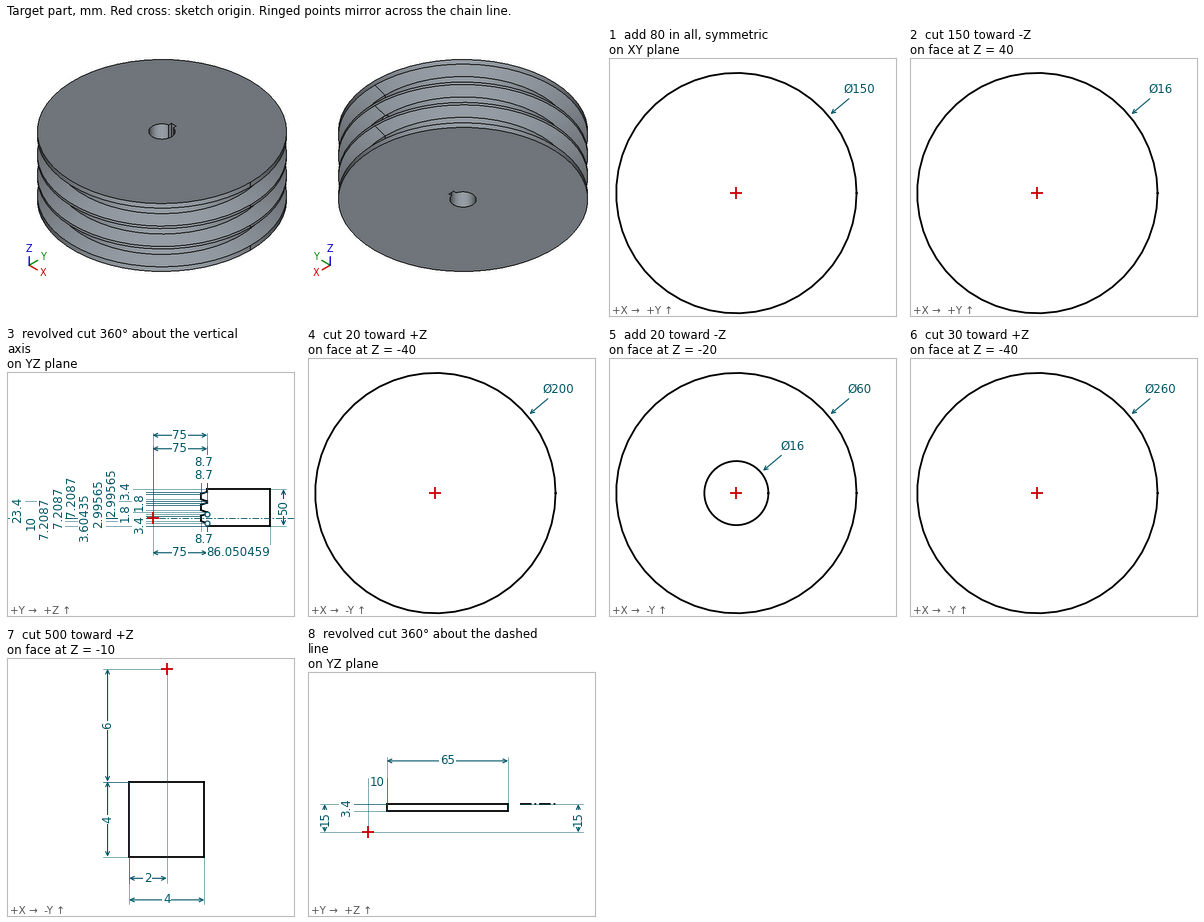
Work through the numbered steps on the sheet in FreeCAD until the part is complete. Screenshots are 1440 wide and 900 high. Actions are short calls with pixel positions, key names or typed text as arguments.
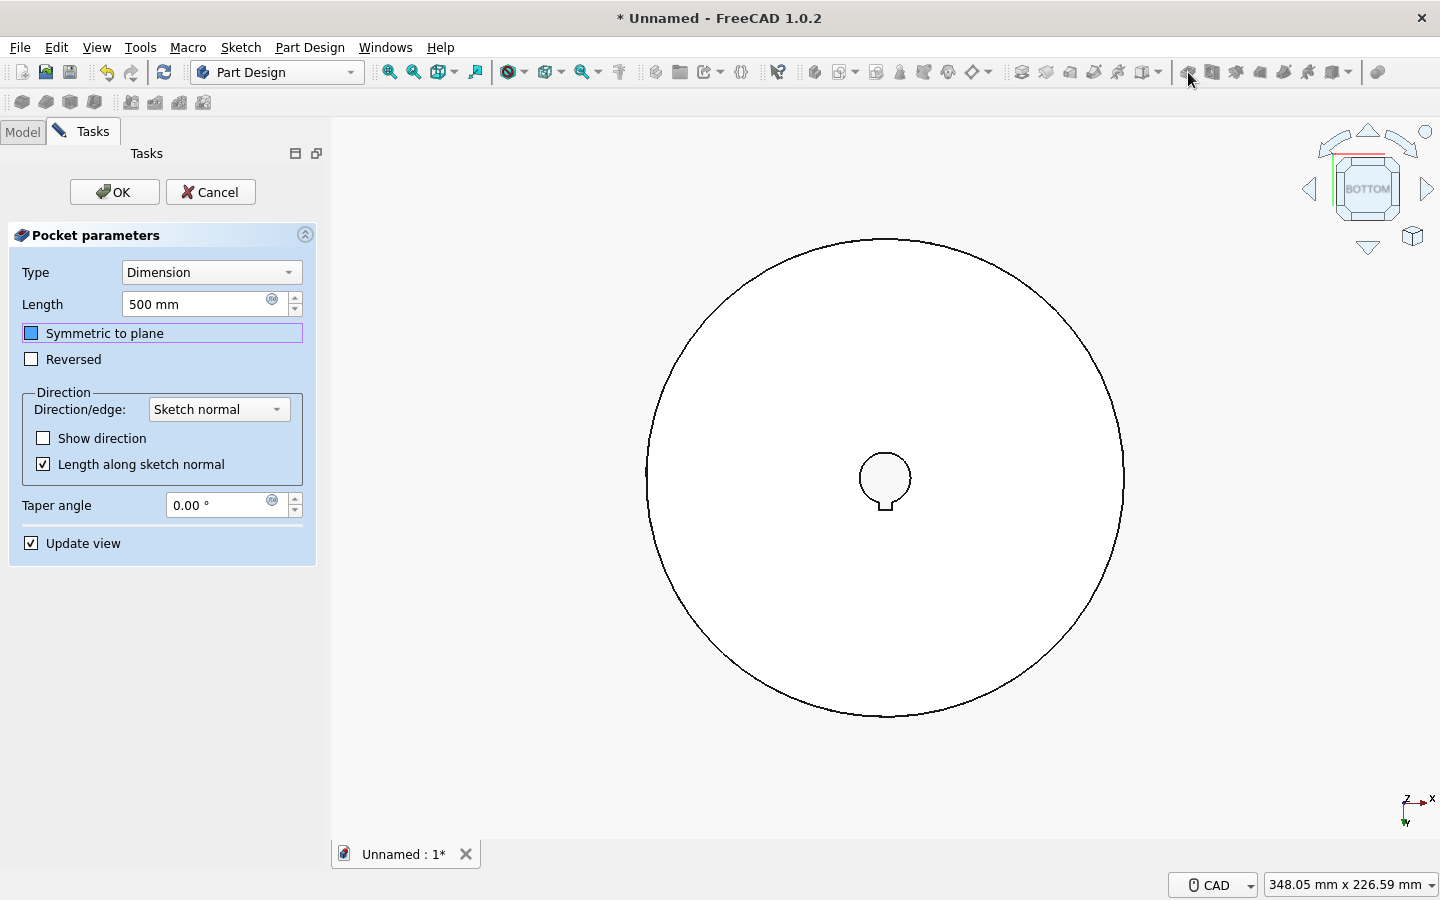
click(115, 192)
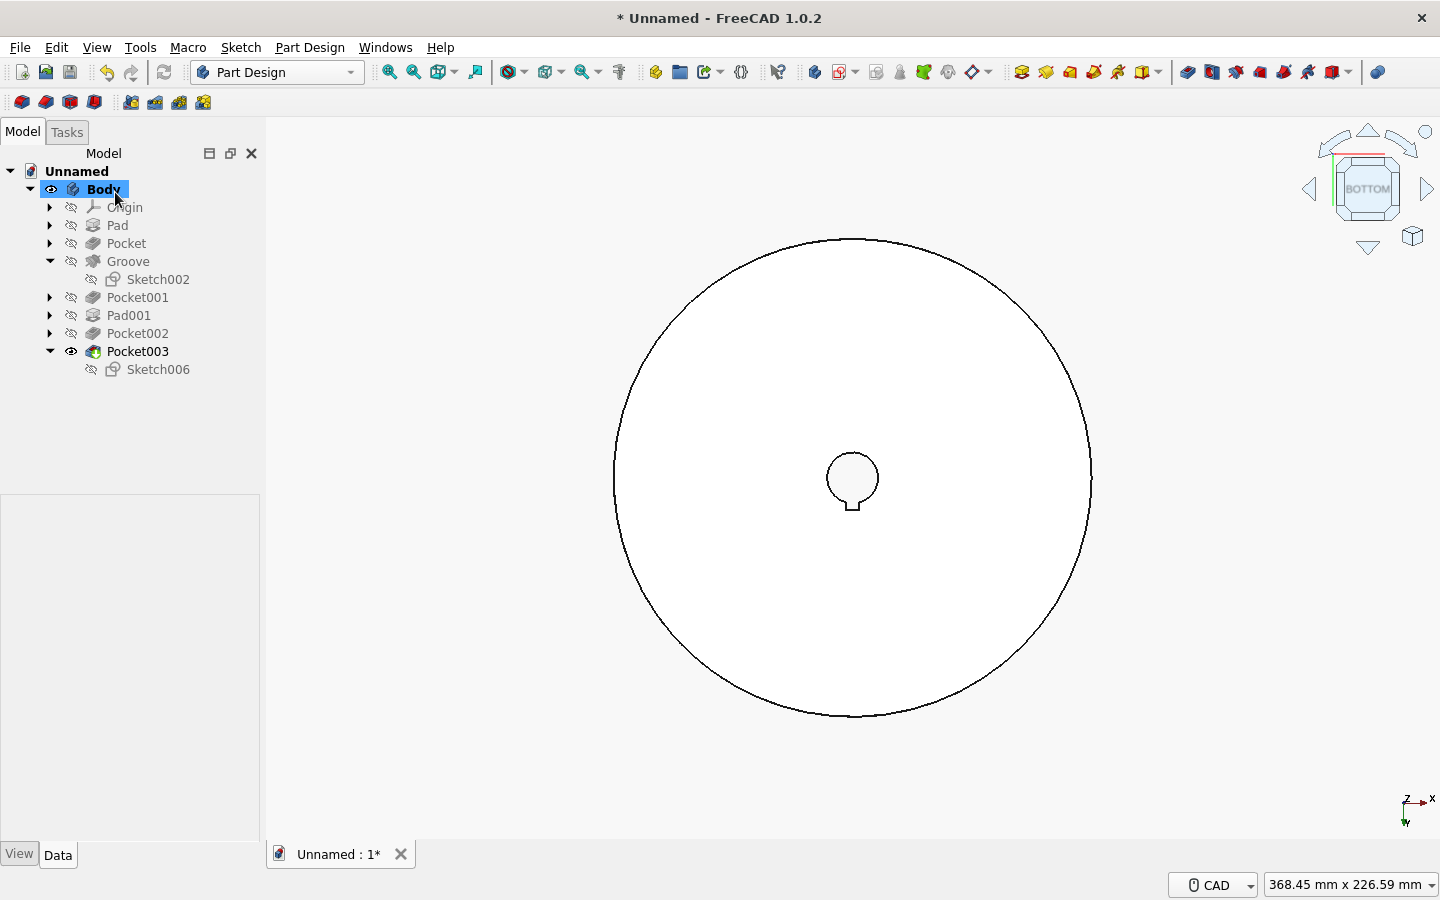
click(840, 72)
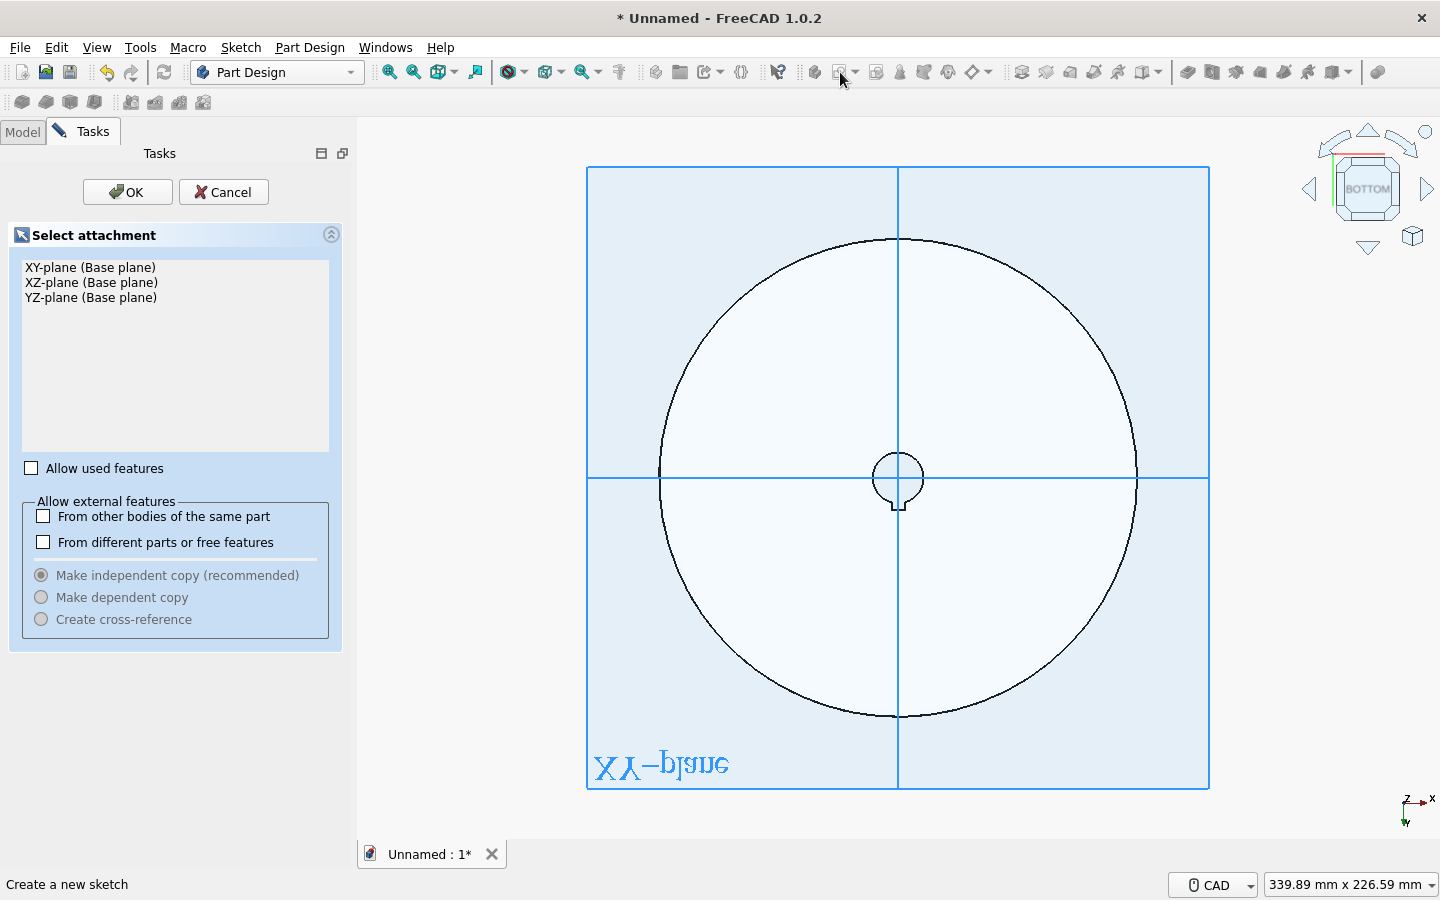
click(82, 298)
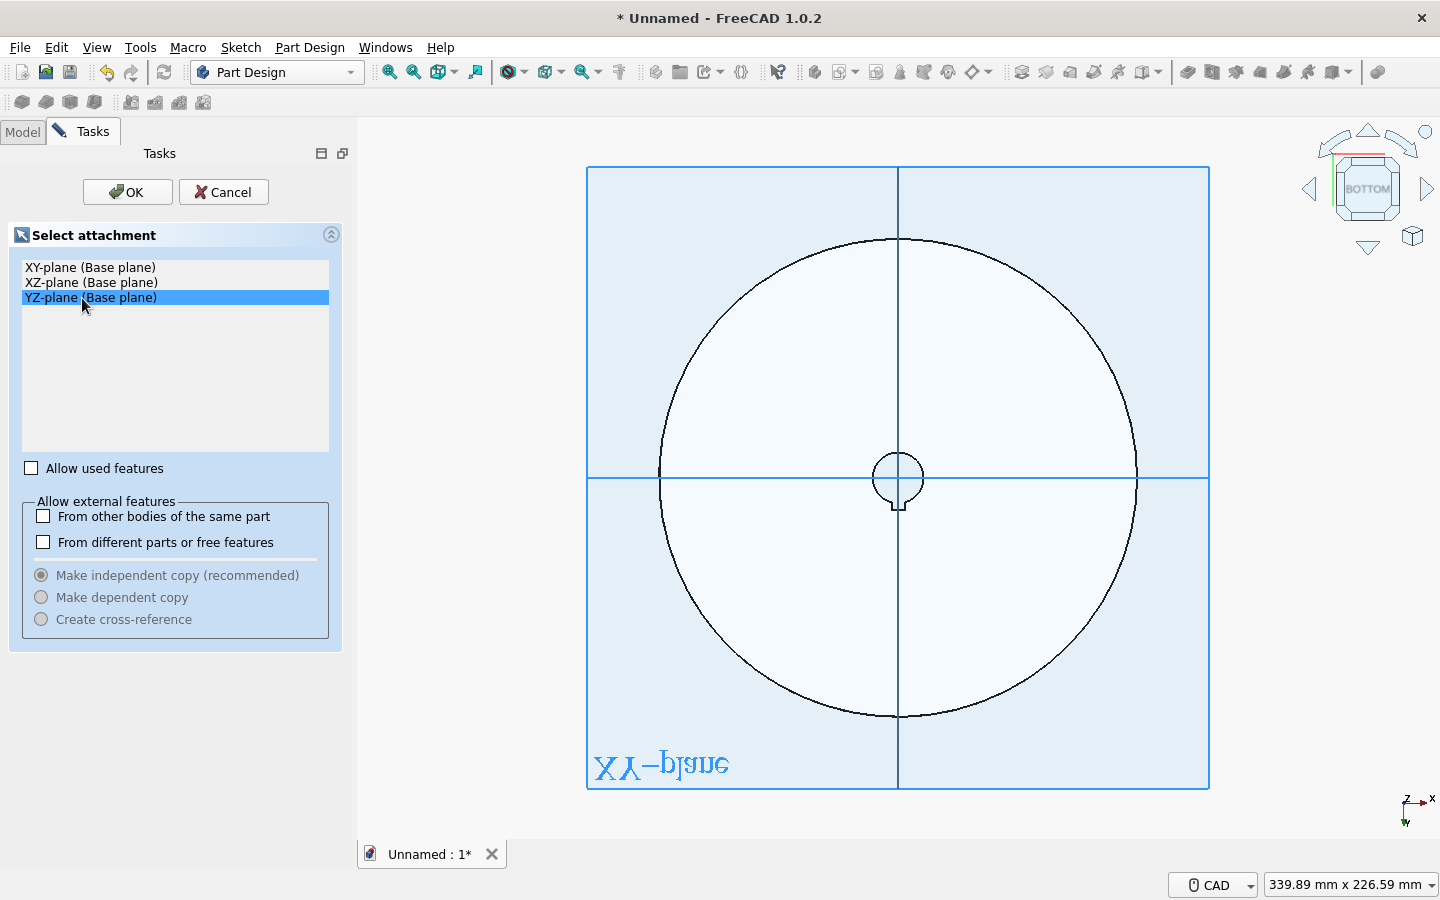
click(128, 192)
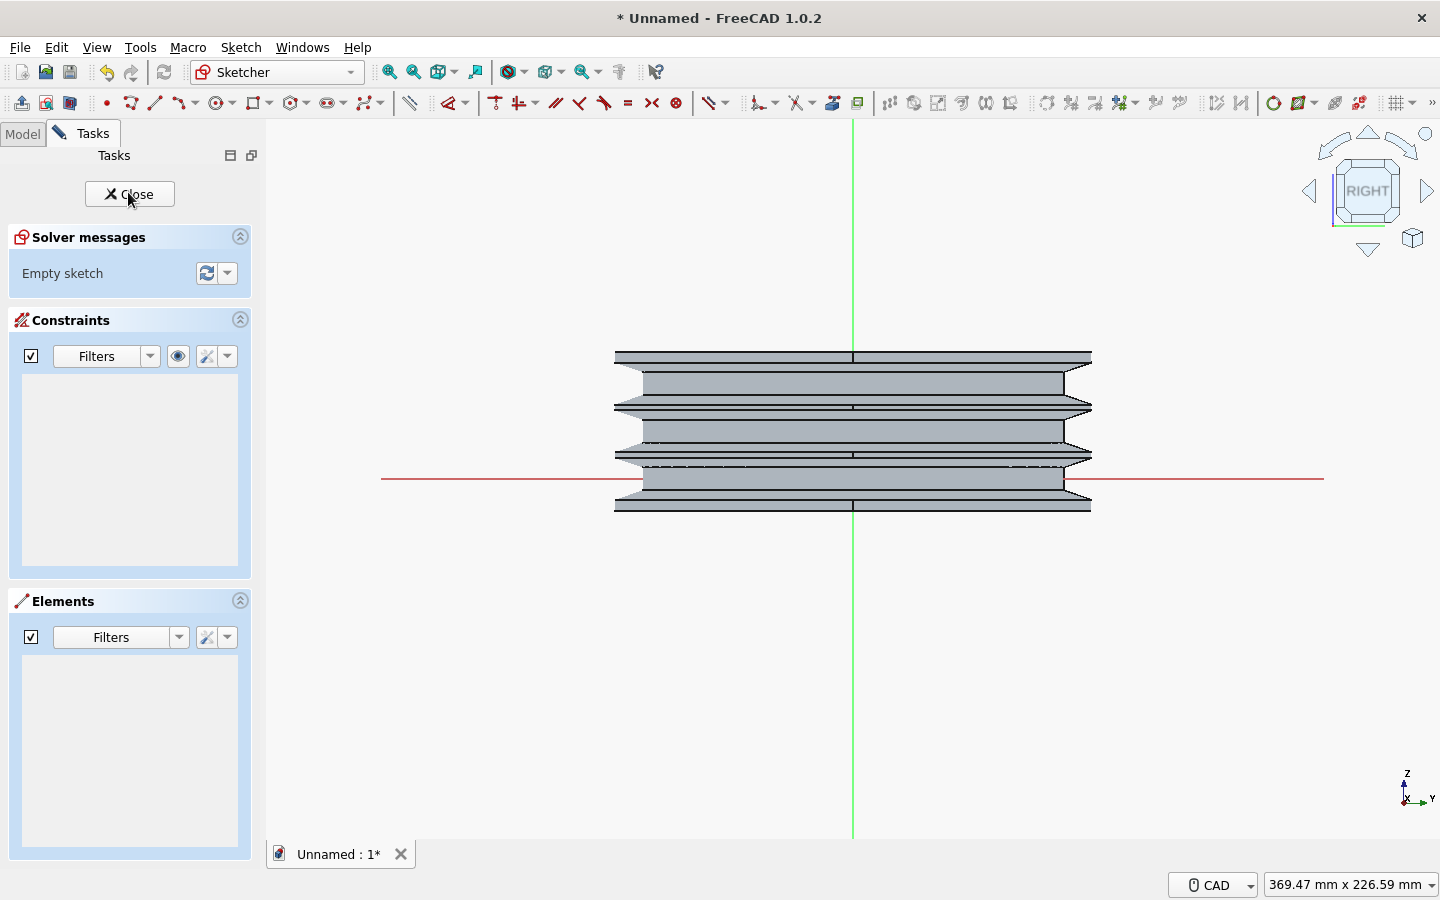
key(q)
key(s)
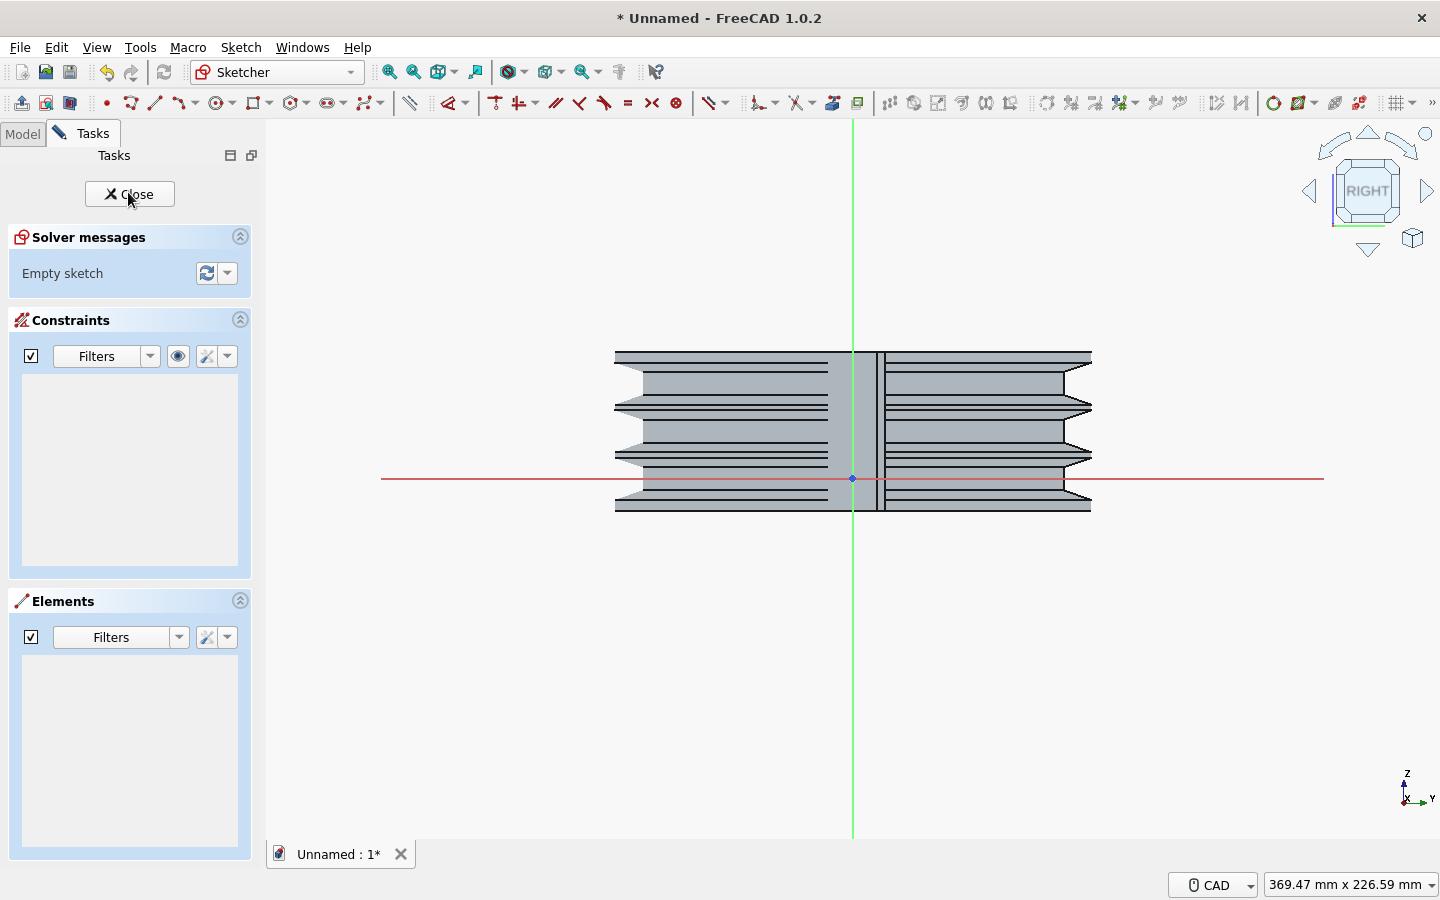
scroll(1200, 436, up, 4)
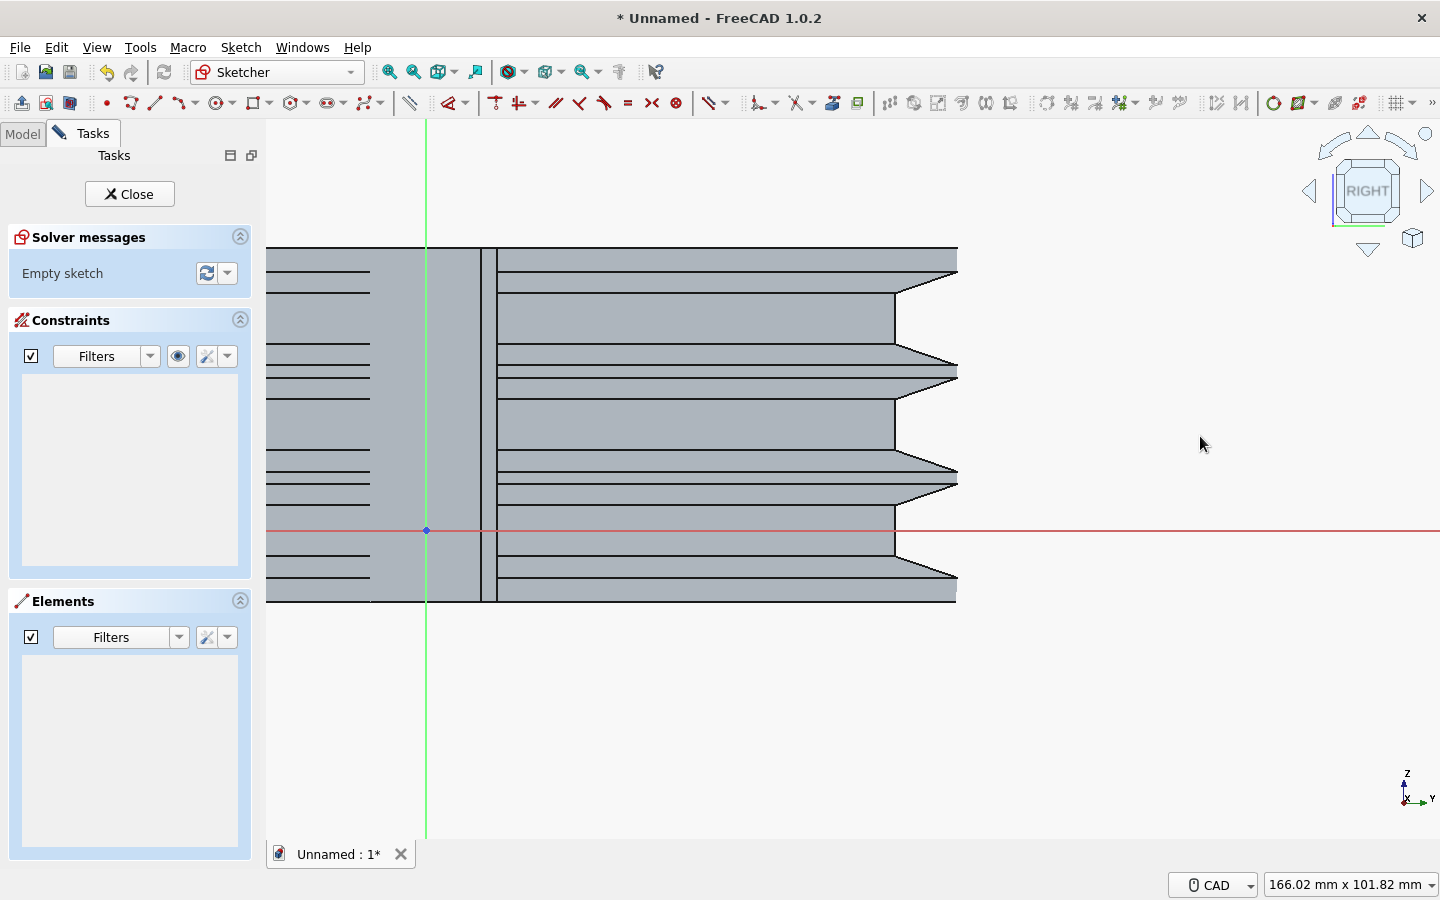
key(g)
key(r)